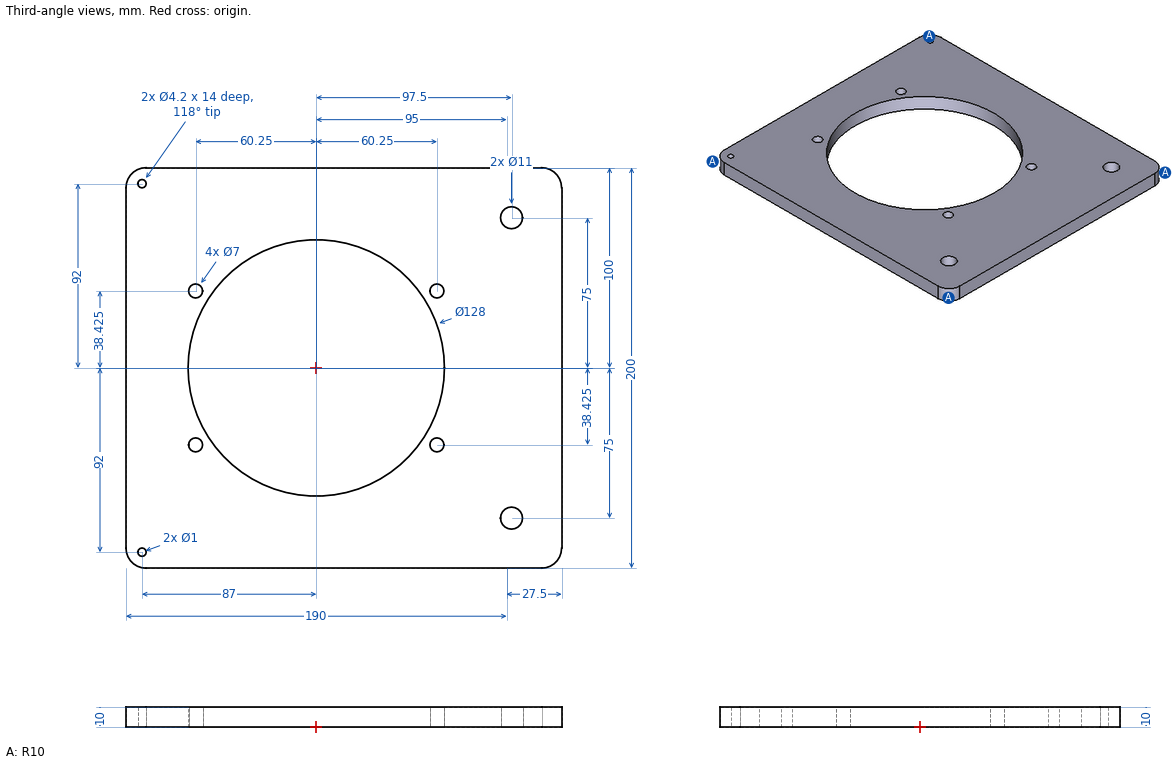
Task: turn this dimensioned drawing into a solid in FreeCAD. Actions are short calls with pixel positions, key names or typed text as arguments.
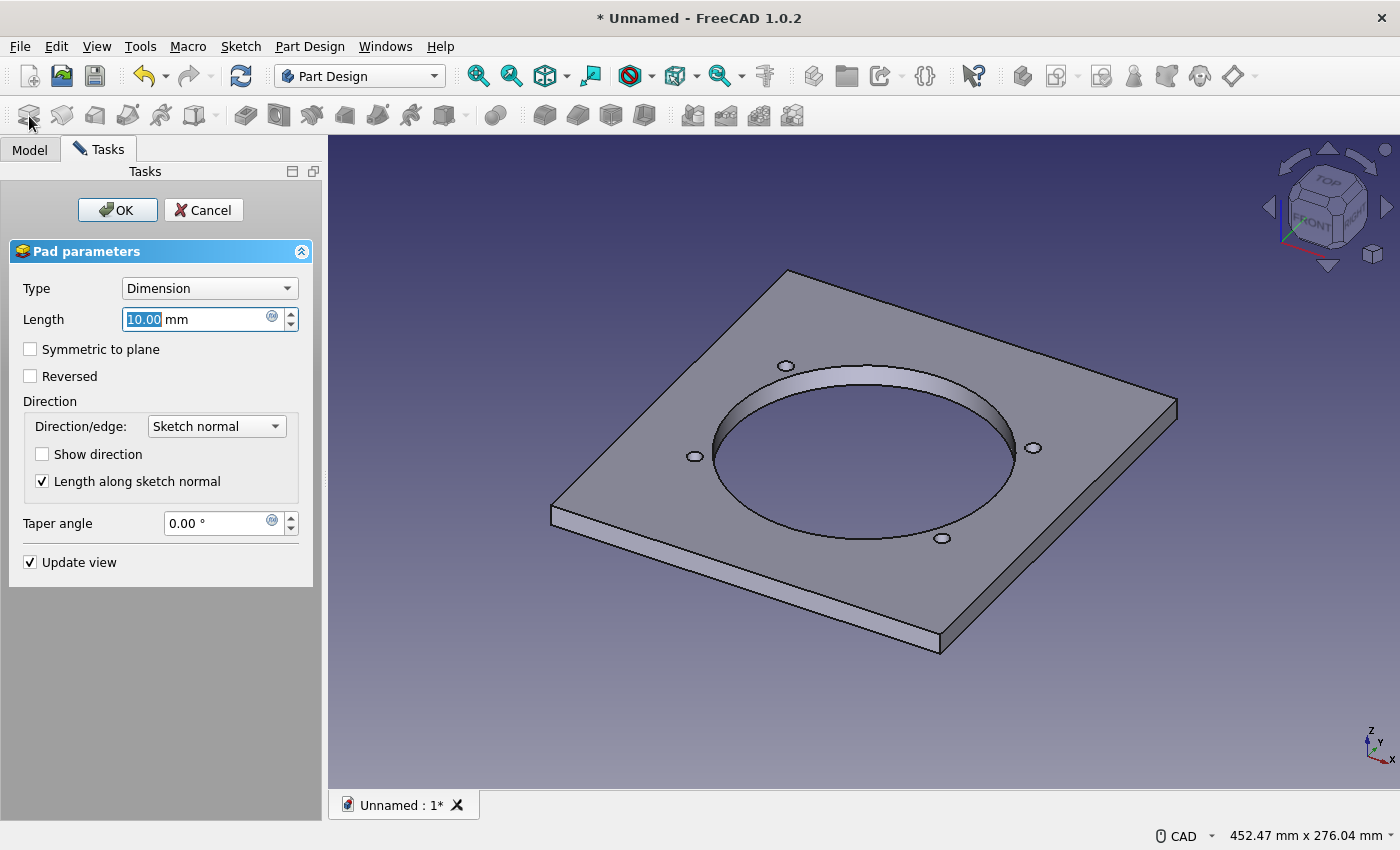
text(10)
key(Tab)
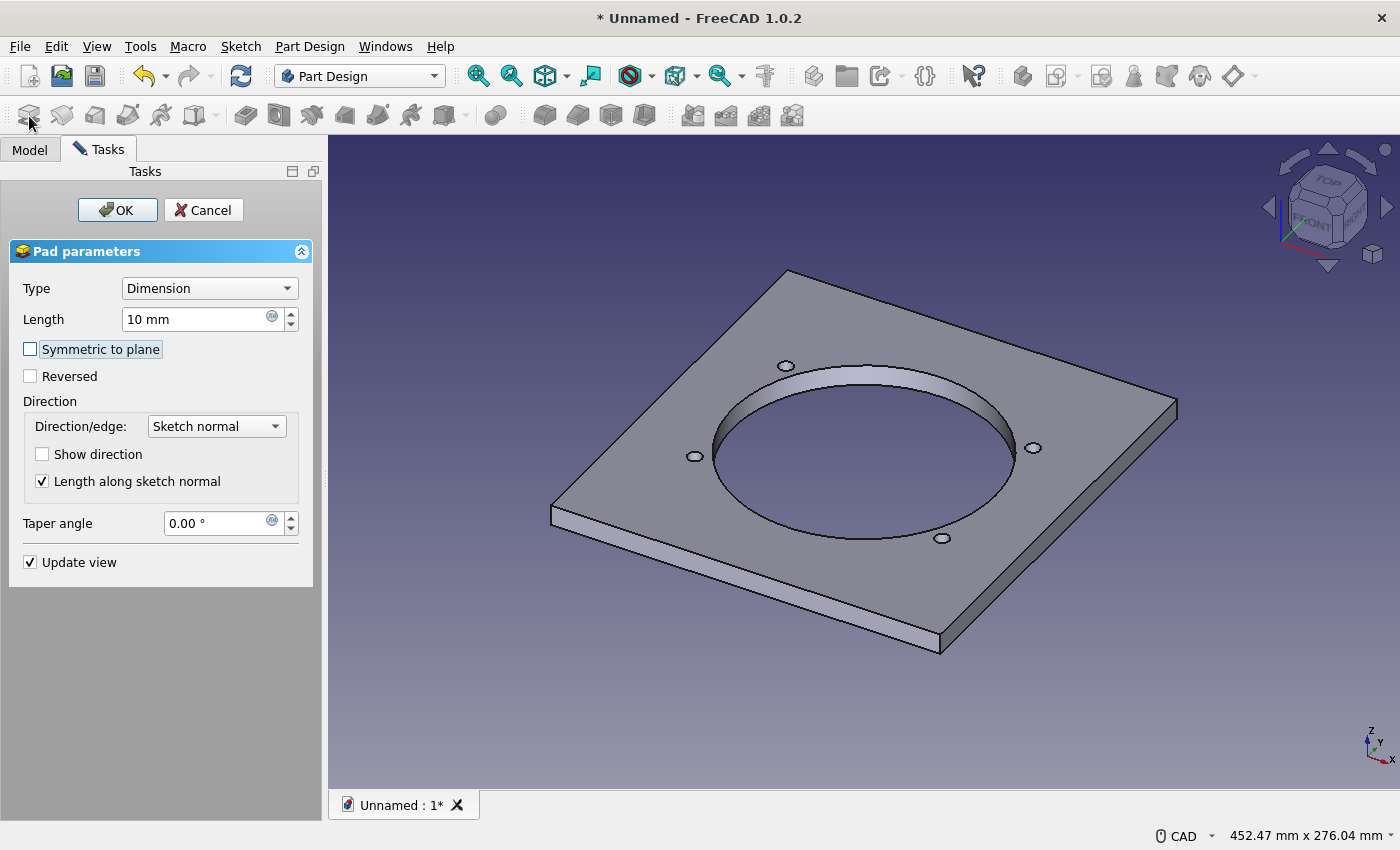
click(31, 376)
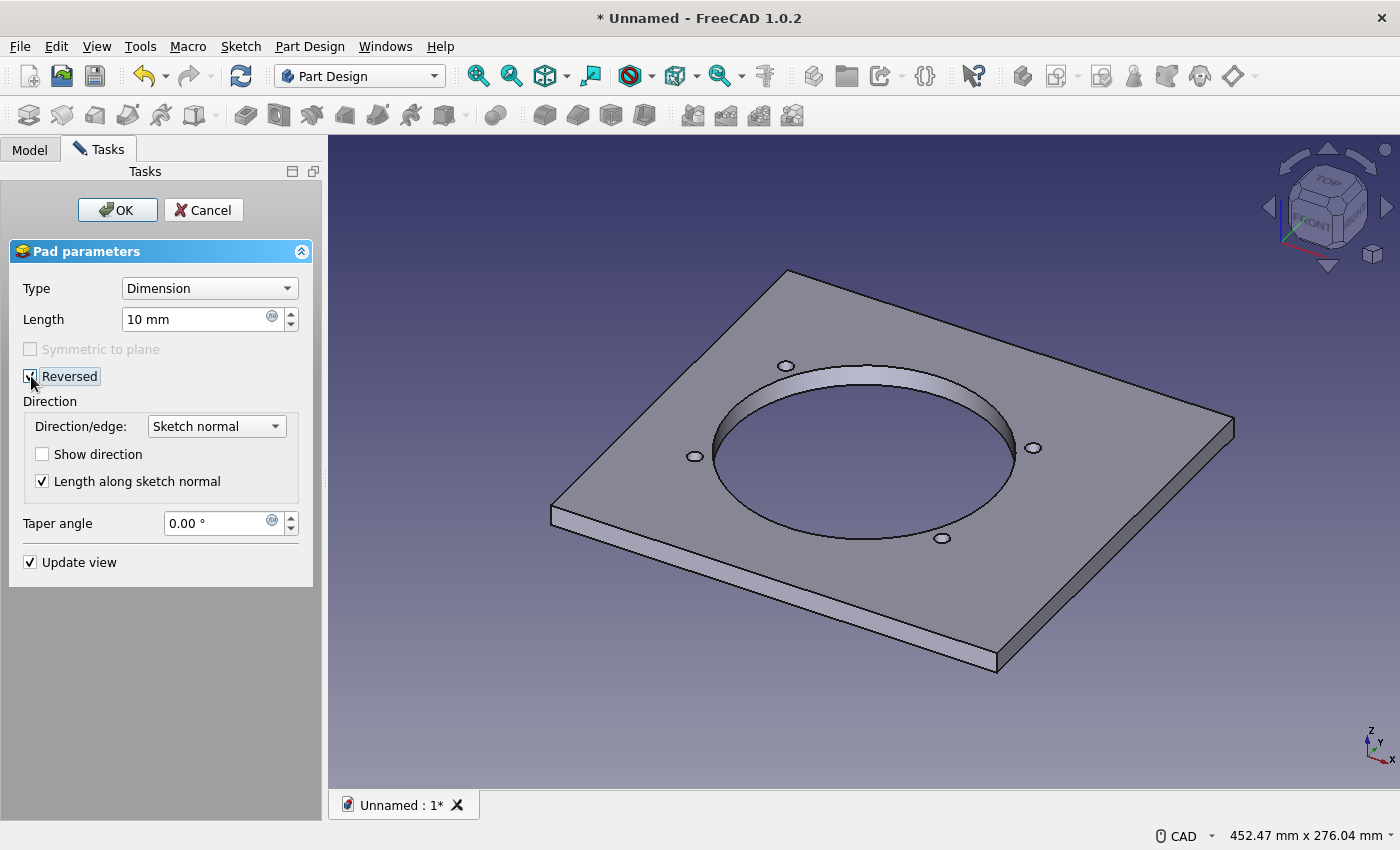
click(118, 210)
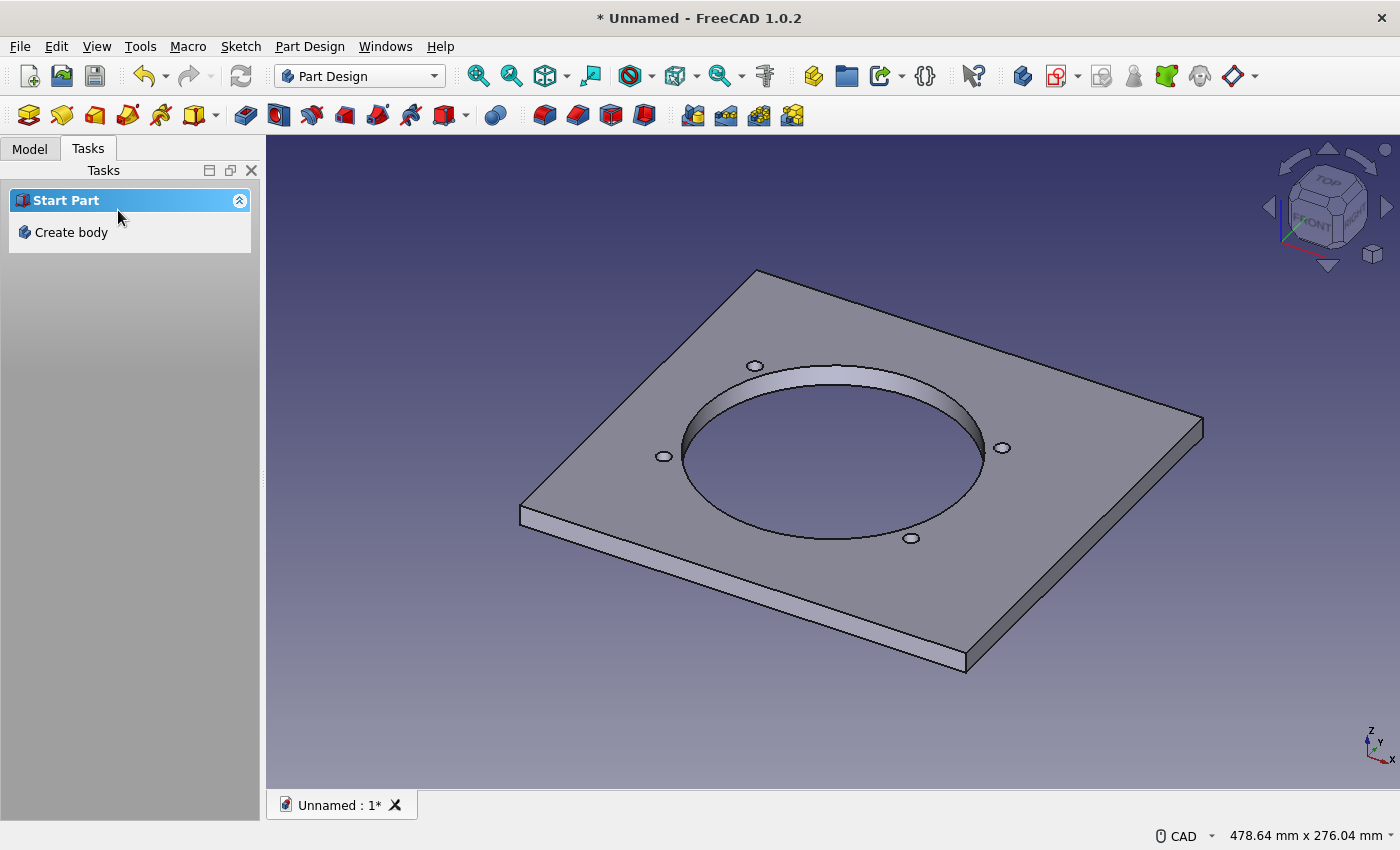
click(921, 570)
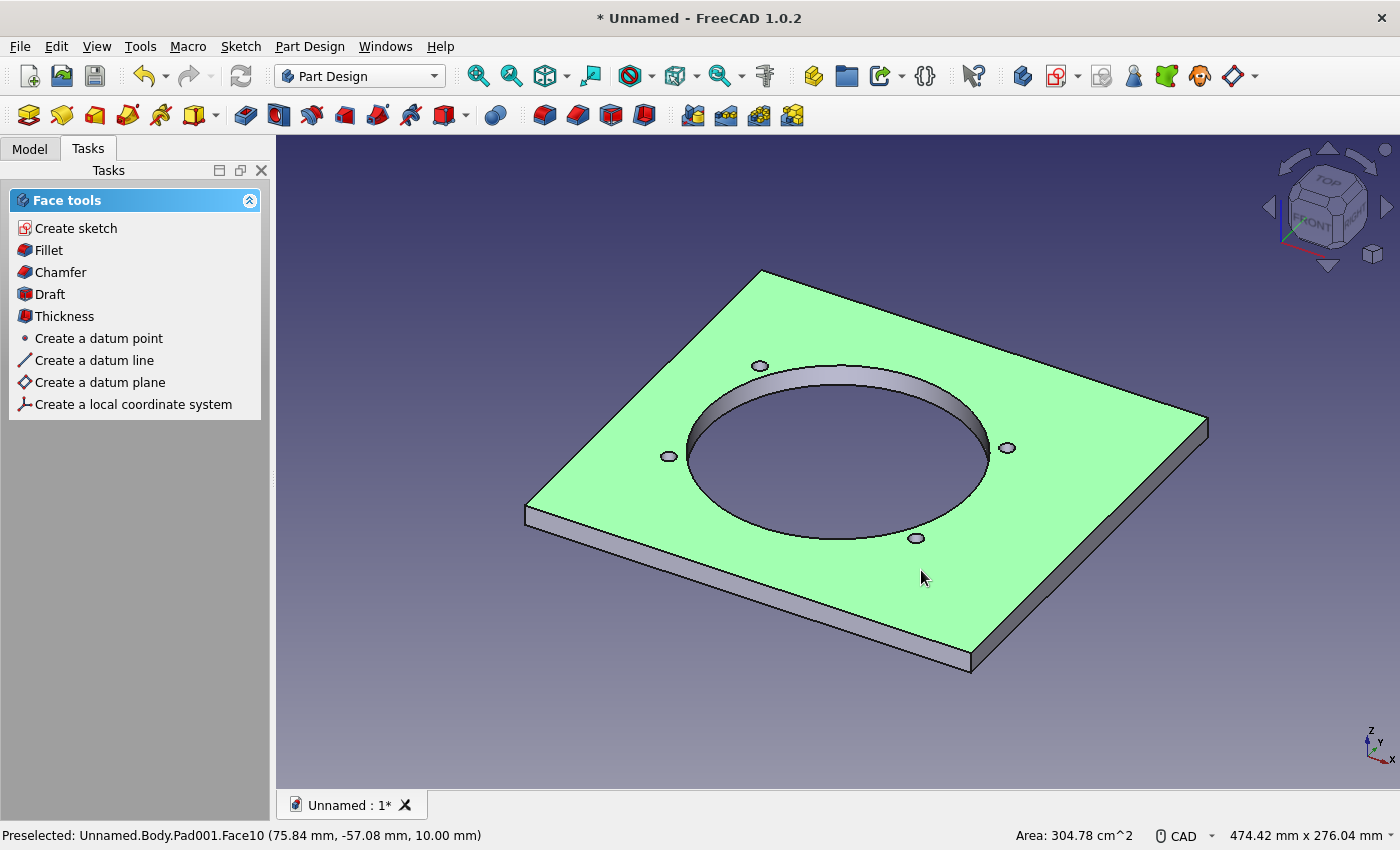
click(1056, 76)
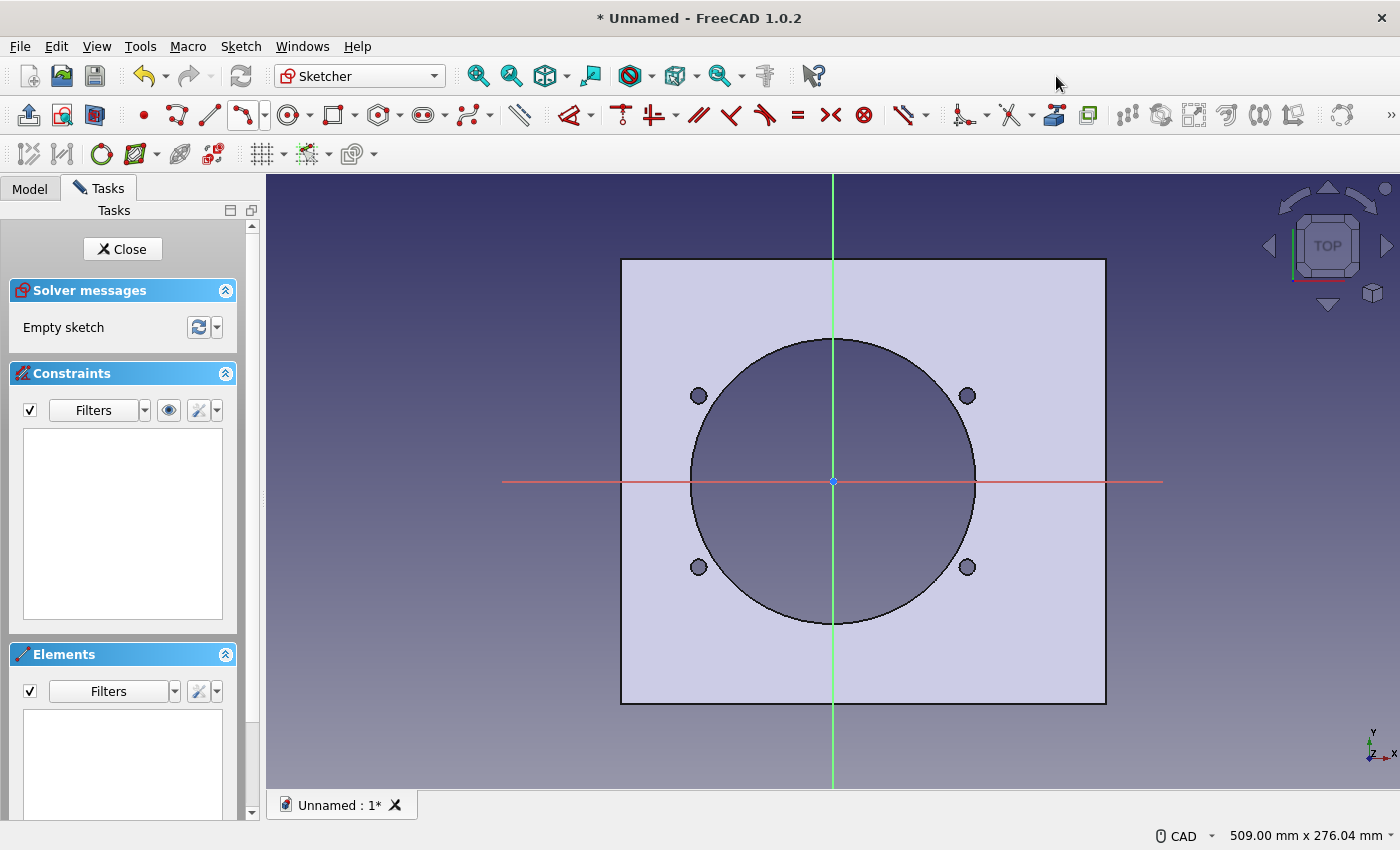
click(288, 116)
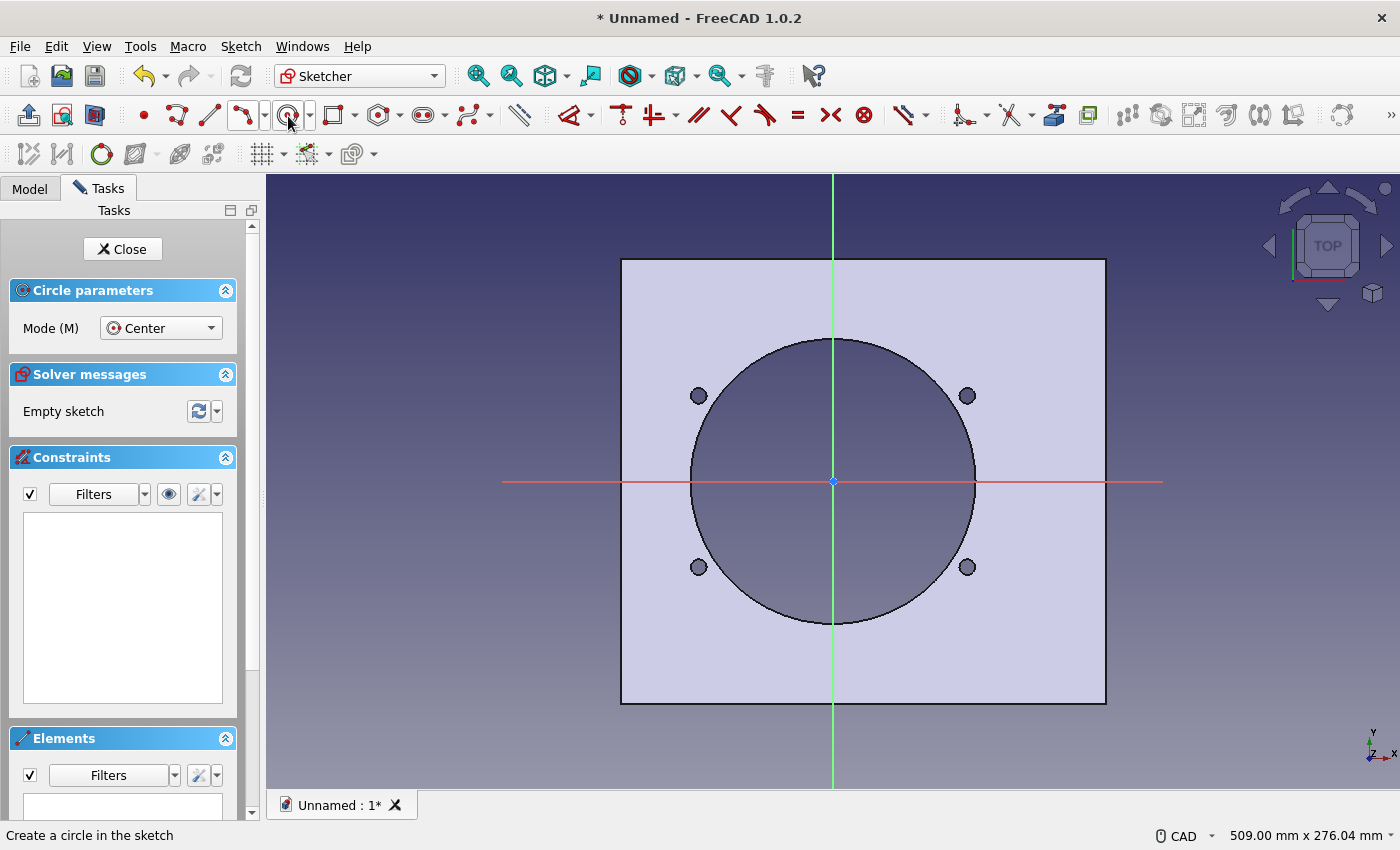
scroll(1050, 314, up, 4)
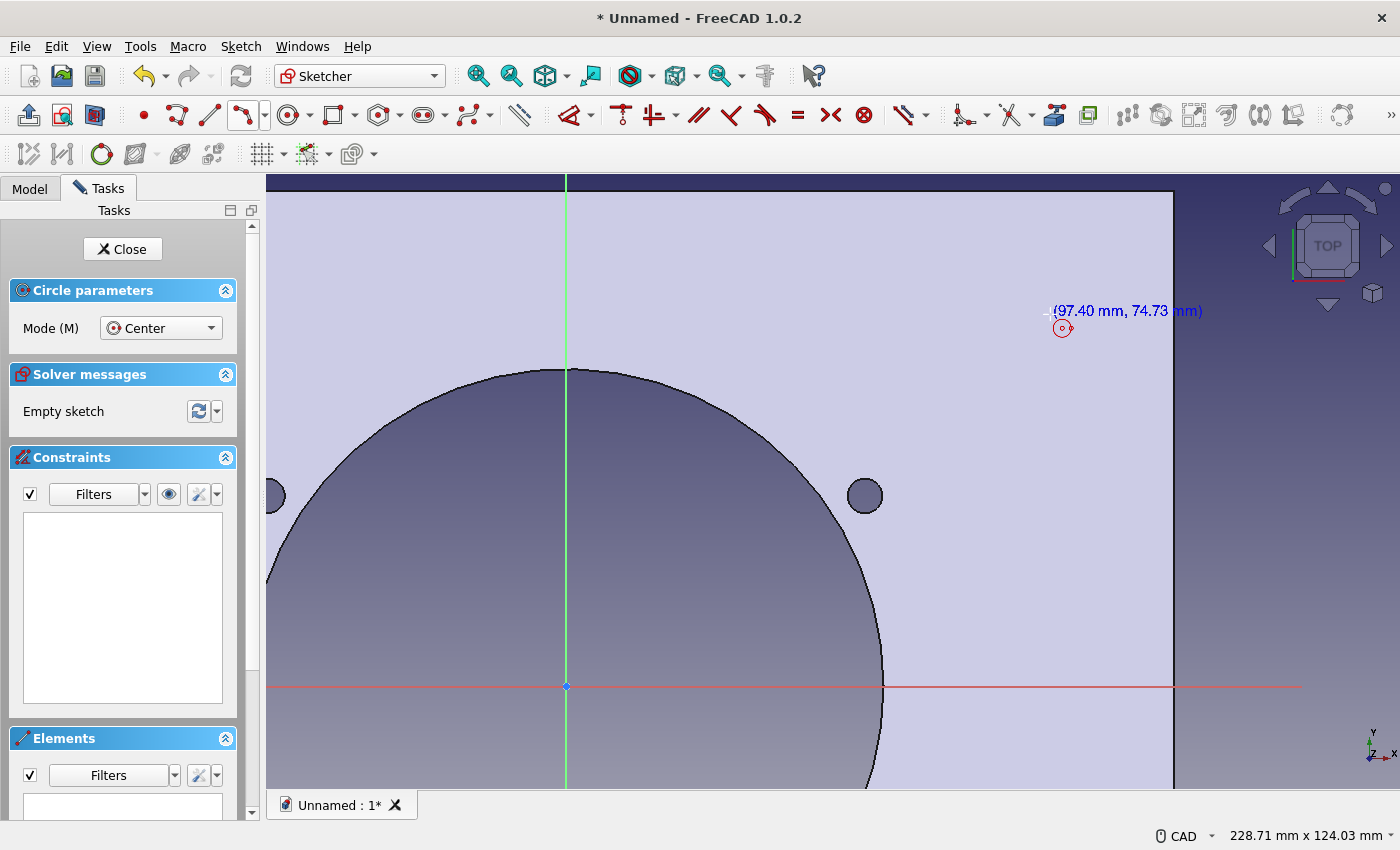
click(1050, 315)
move(1069, 295)